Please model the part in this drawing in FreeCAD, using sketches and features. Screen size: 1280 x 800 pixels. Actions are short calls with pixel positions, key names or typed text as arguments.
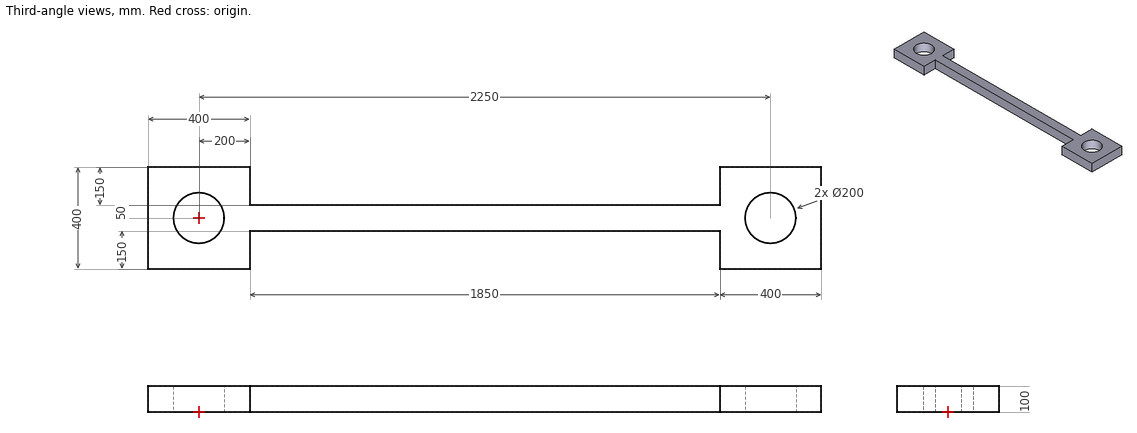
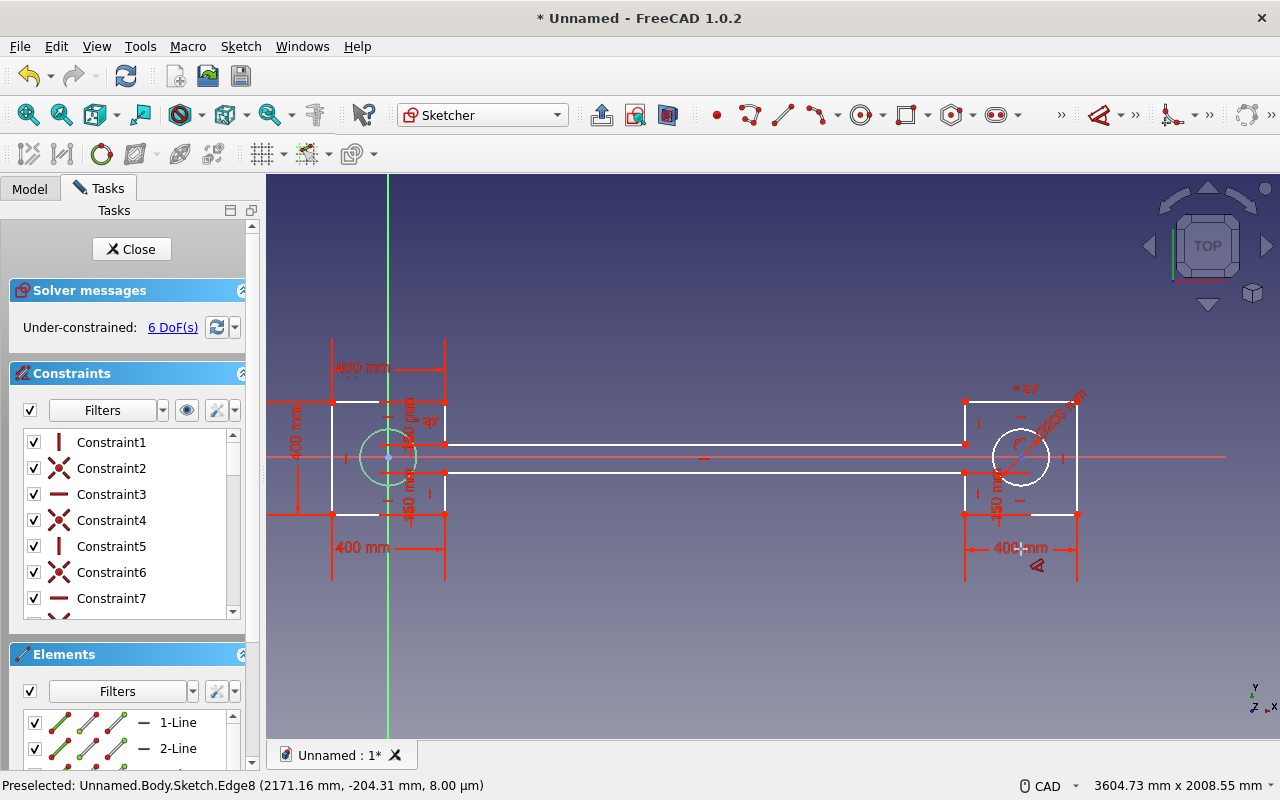
click(1077, 481)
click(1111, 484)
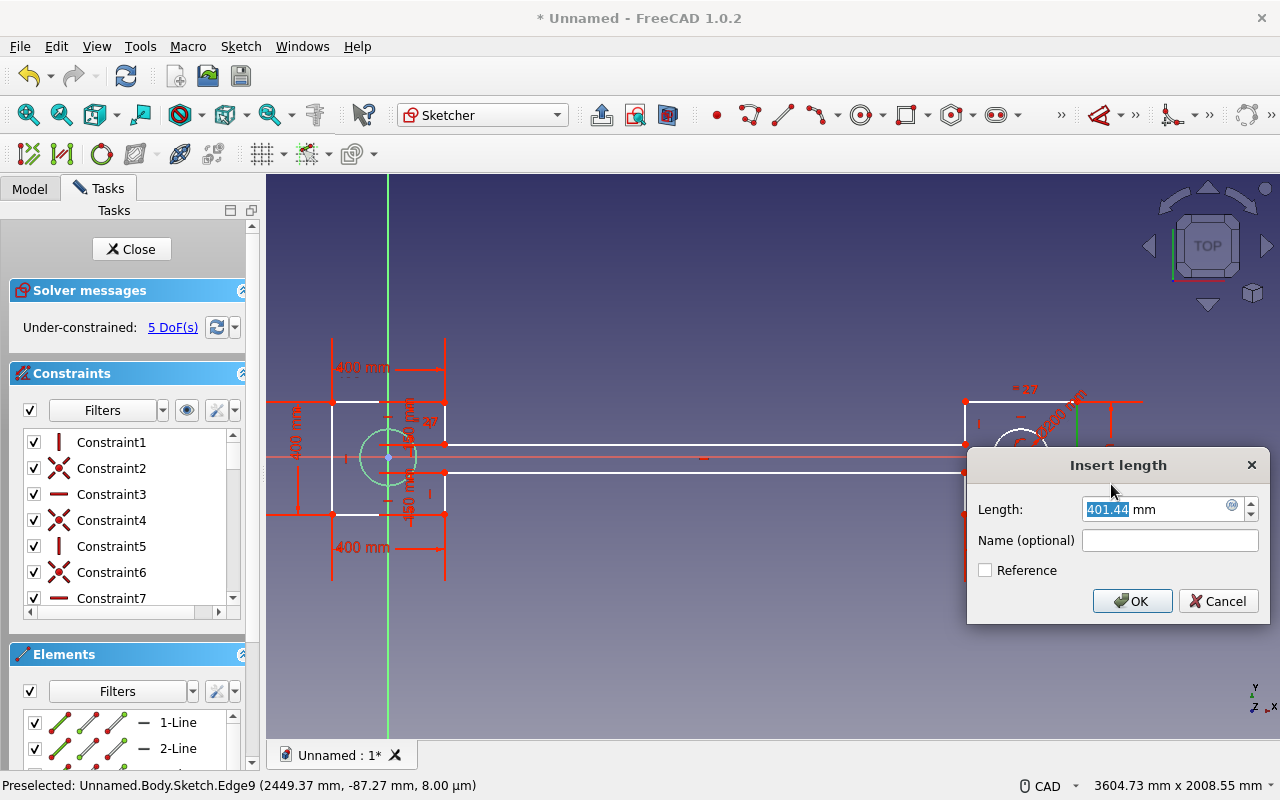
text(400)
key(Return)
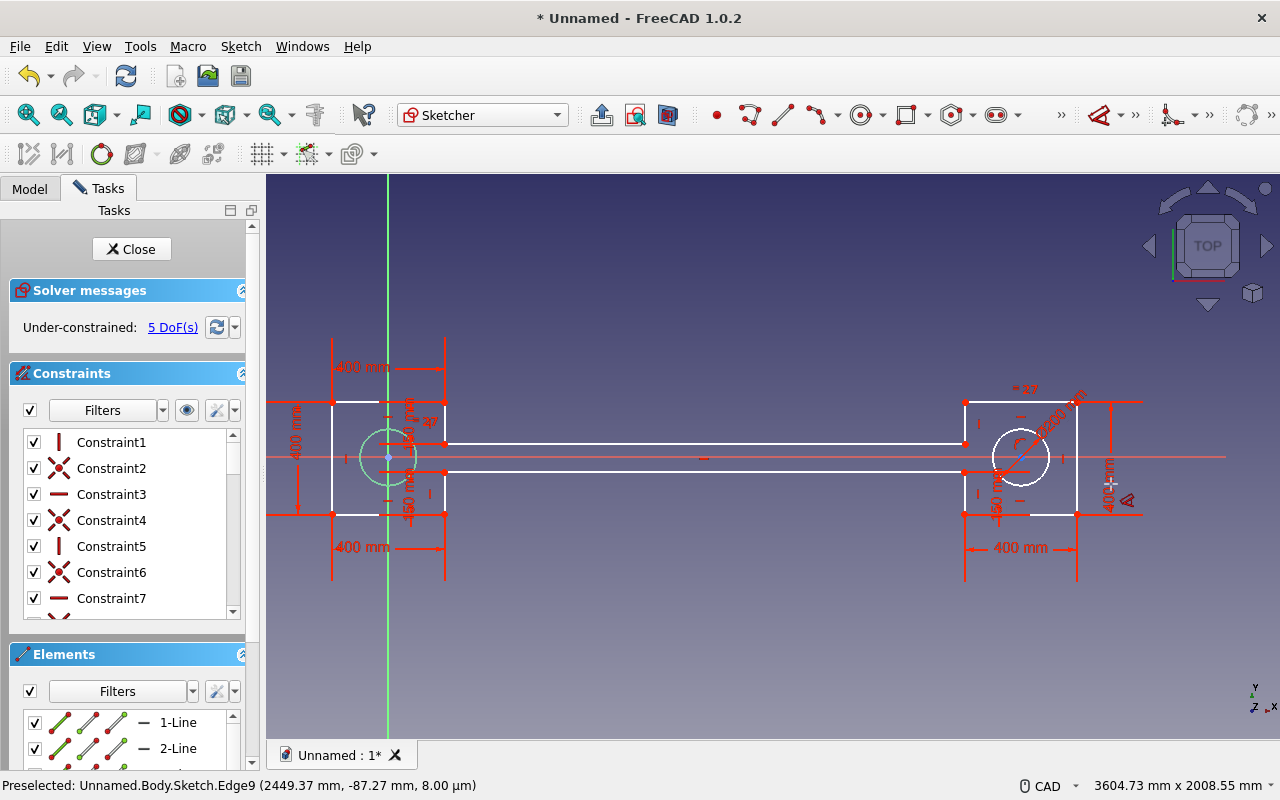
click(1044, 402)
click(1021, 368)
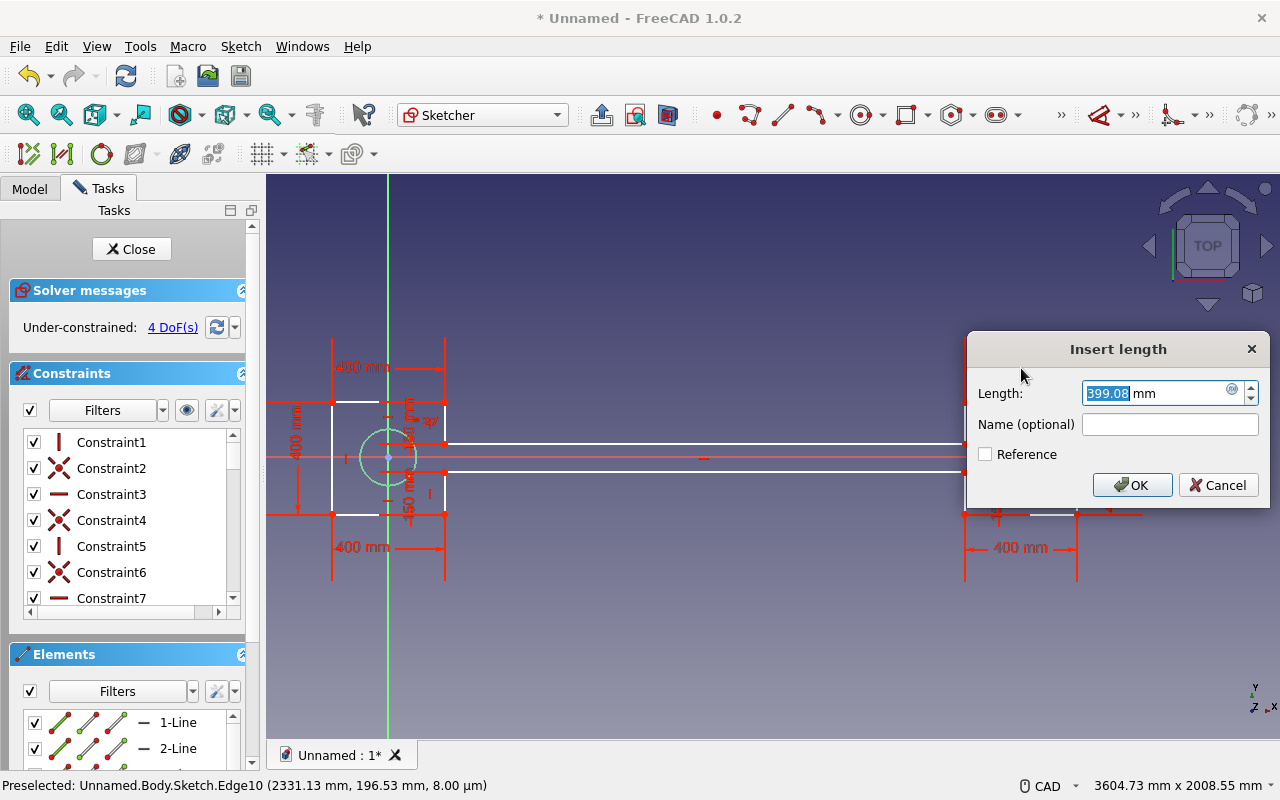
text(400)
key(Return)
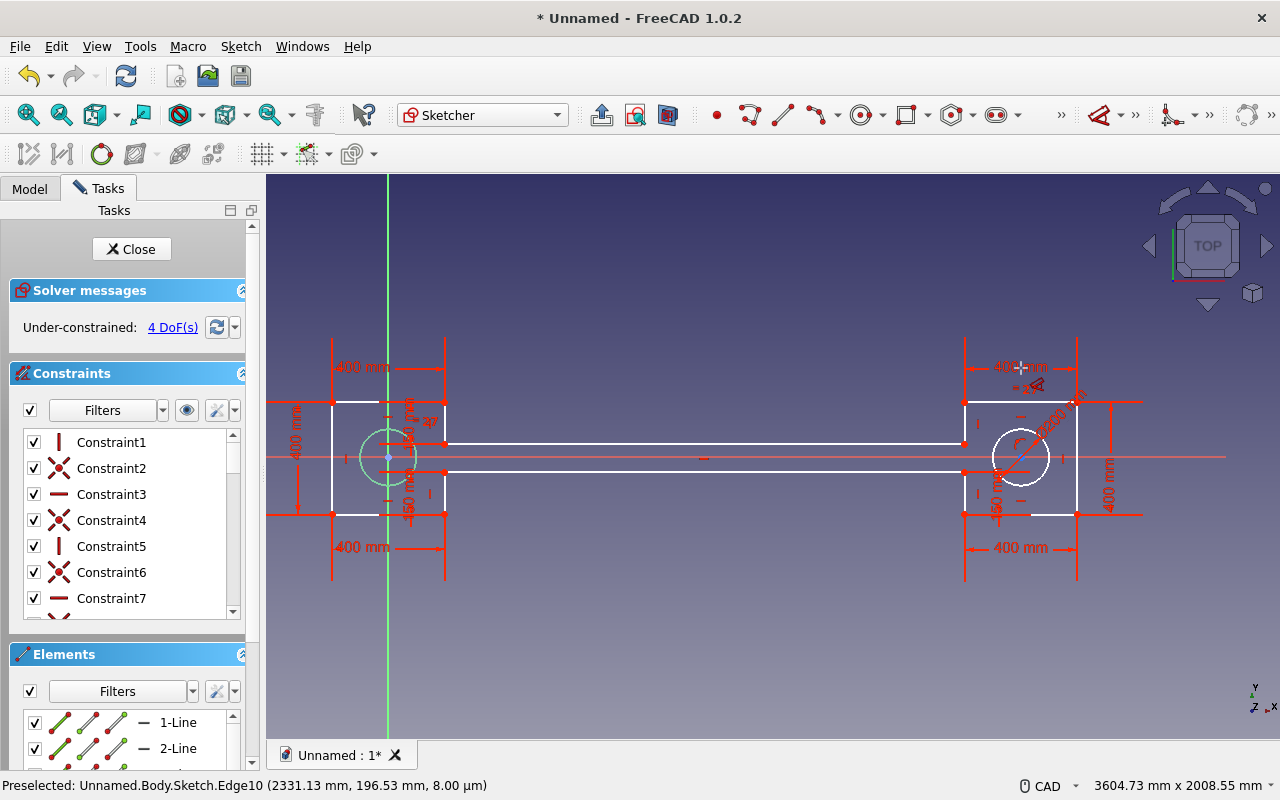
scroll(445, 444, up, 6)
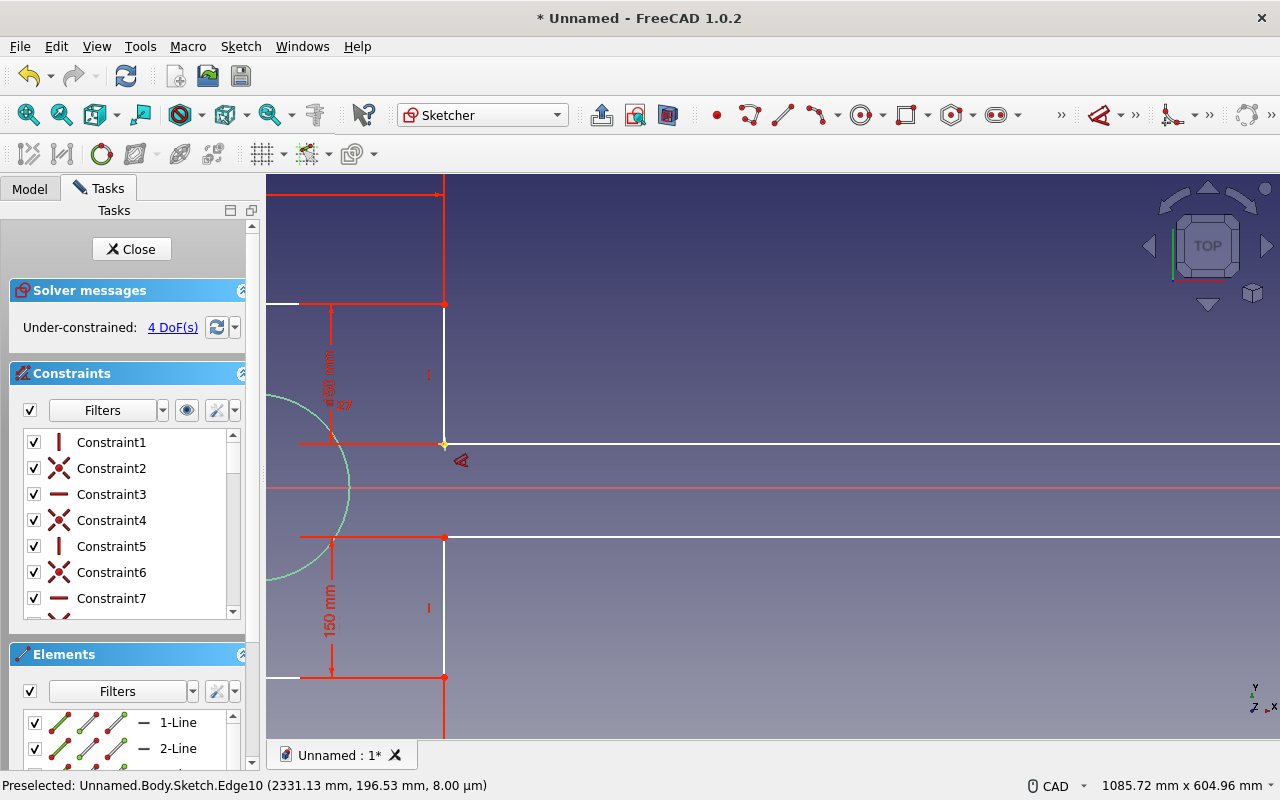
click(444, 444)
click(478, 466)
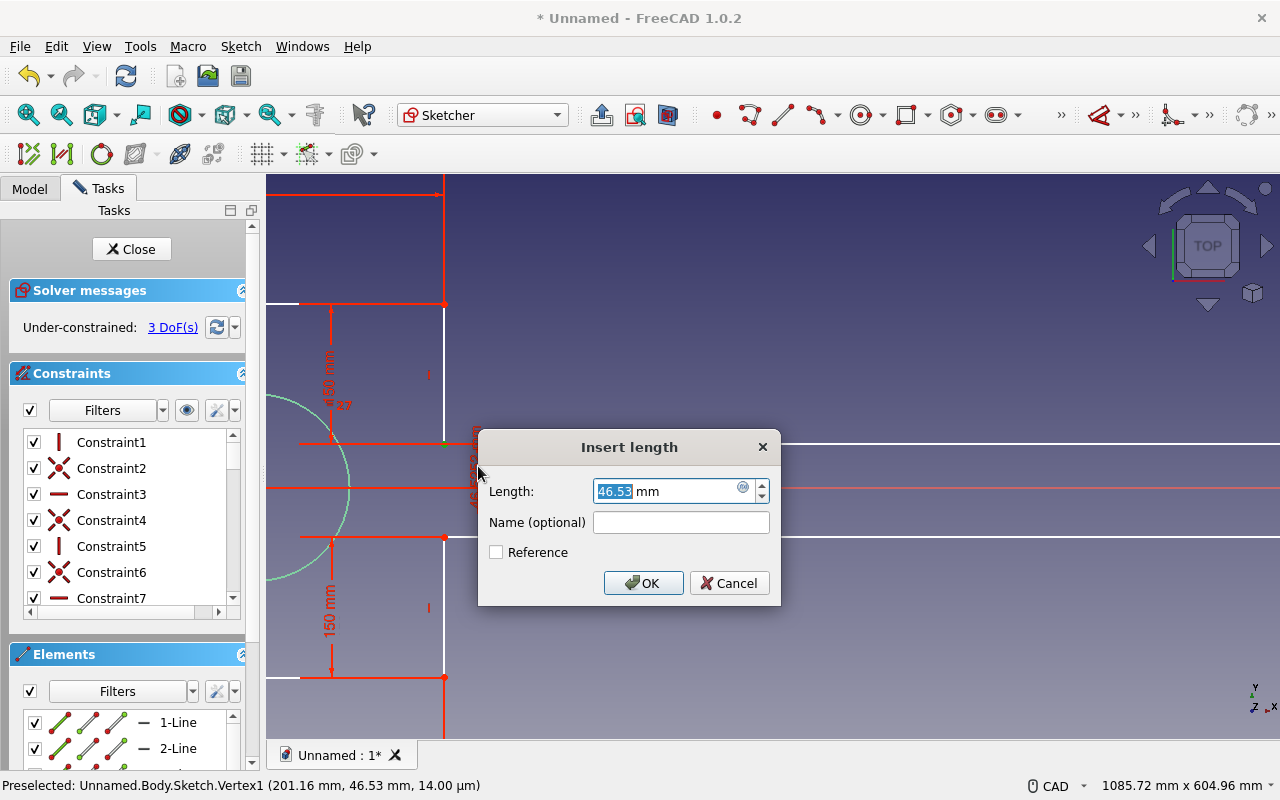
text(50)
key(Return)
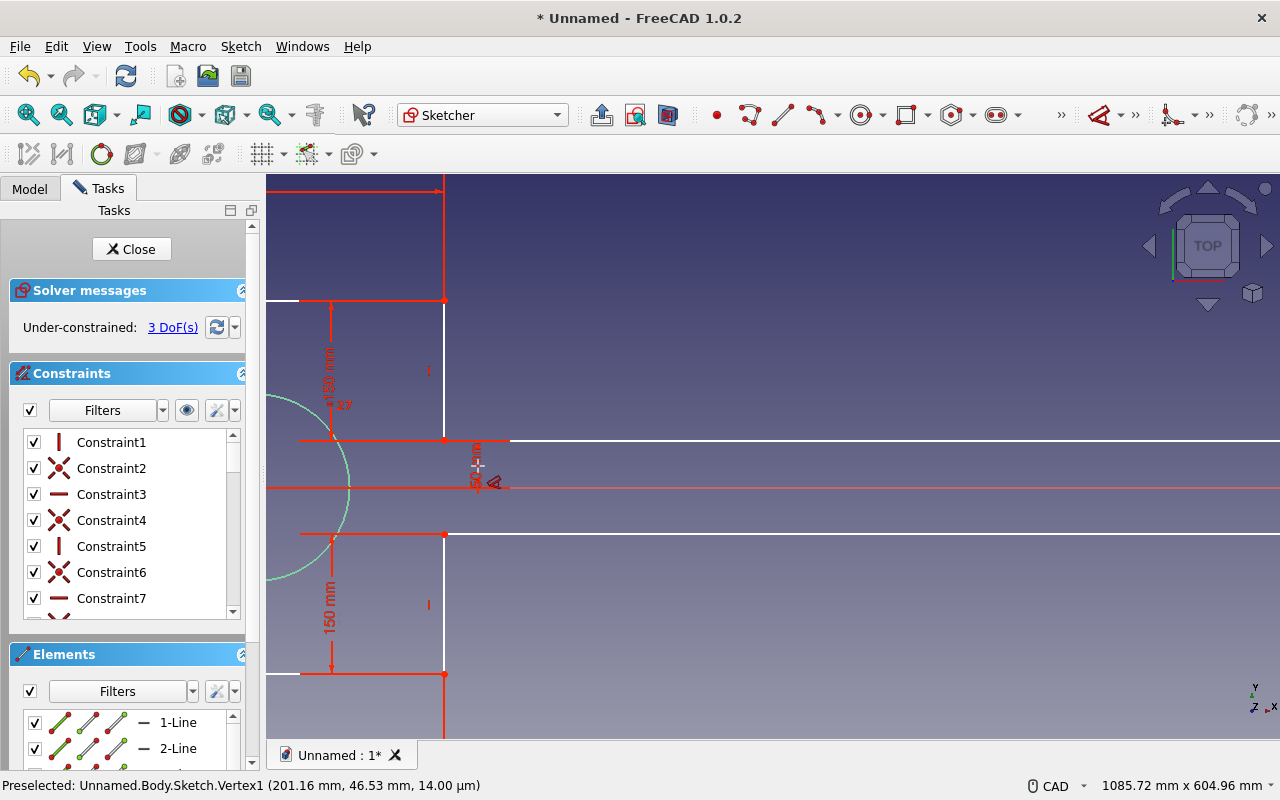
click(962, 534)
click(780, 568)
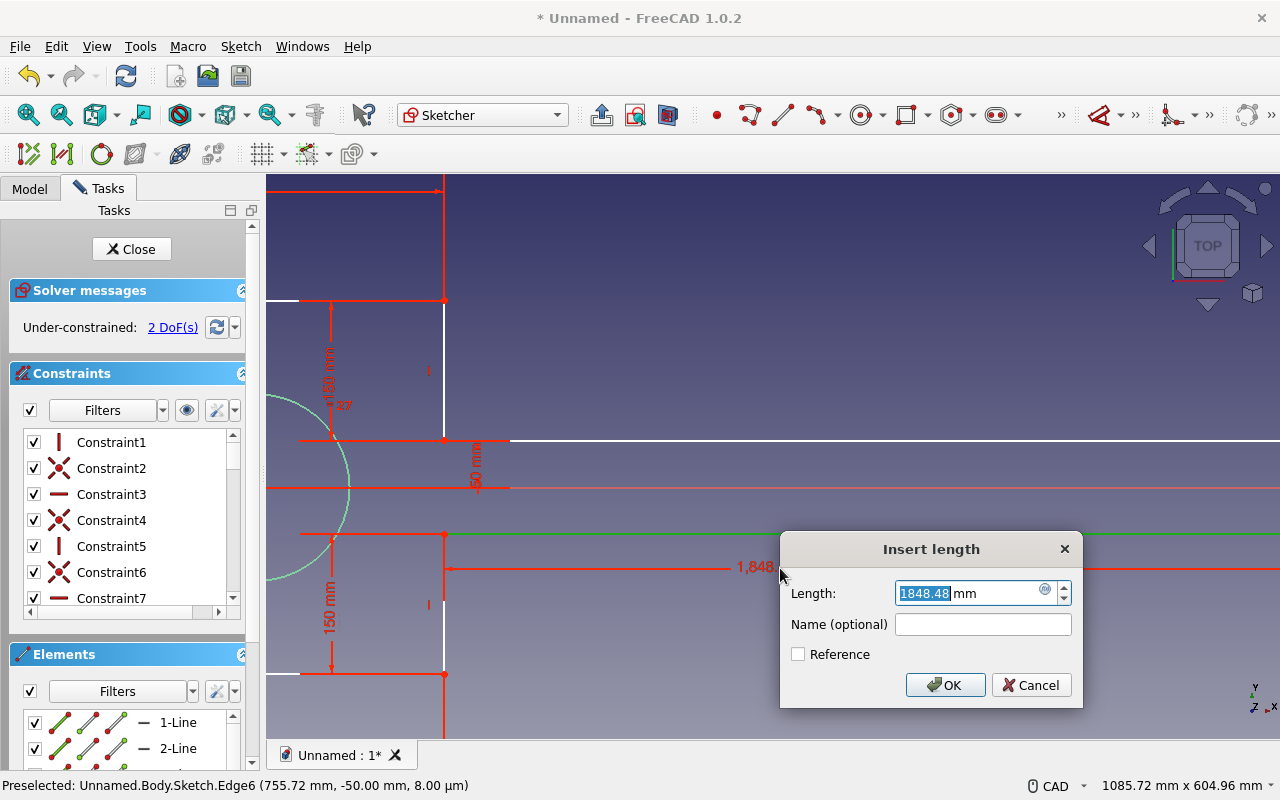
text(1850)
key(Return)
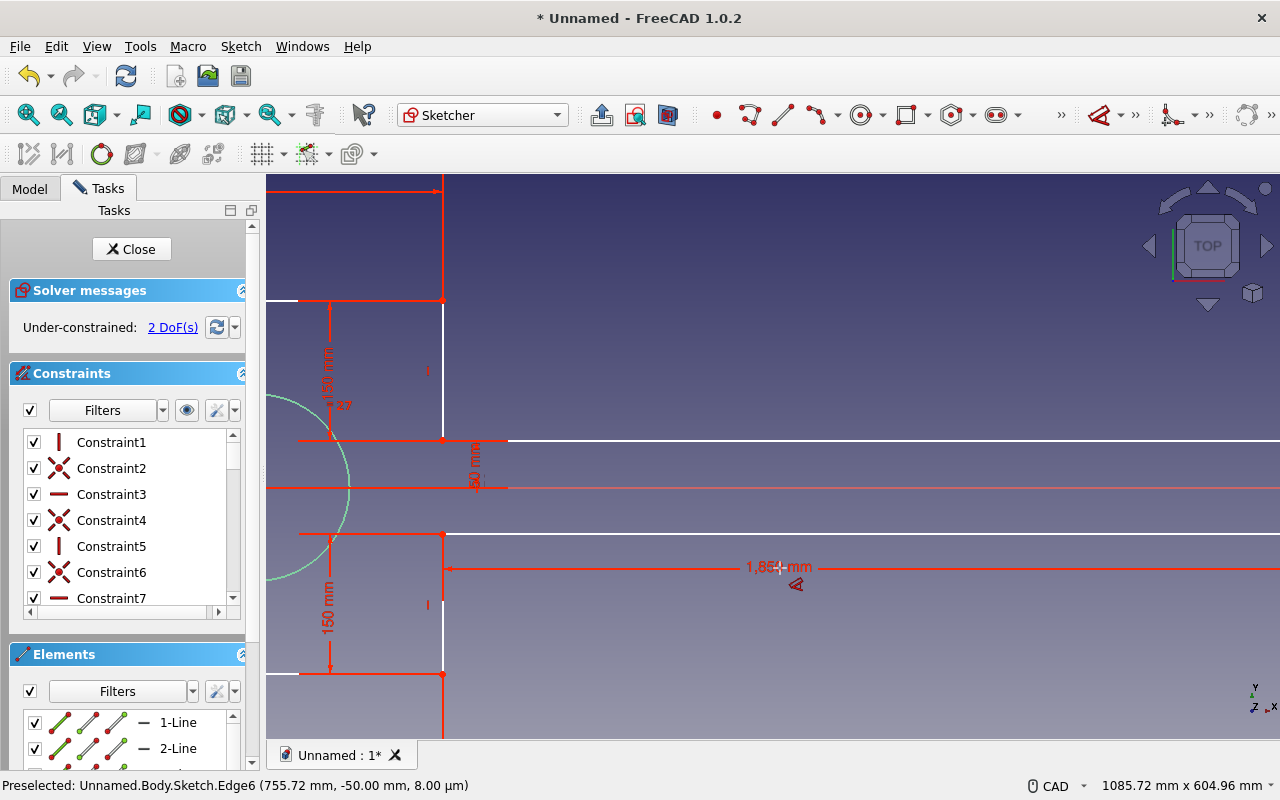
click(443, 441)
click(368, 407)